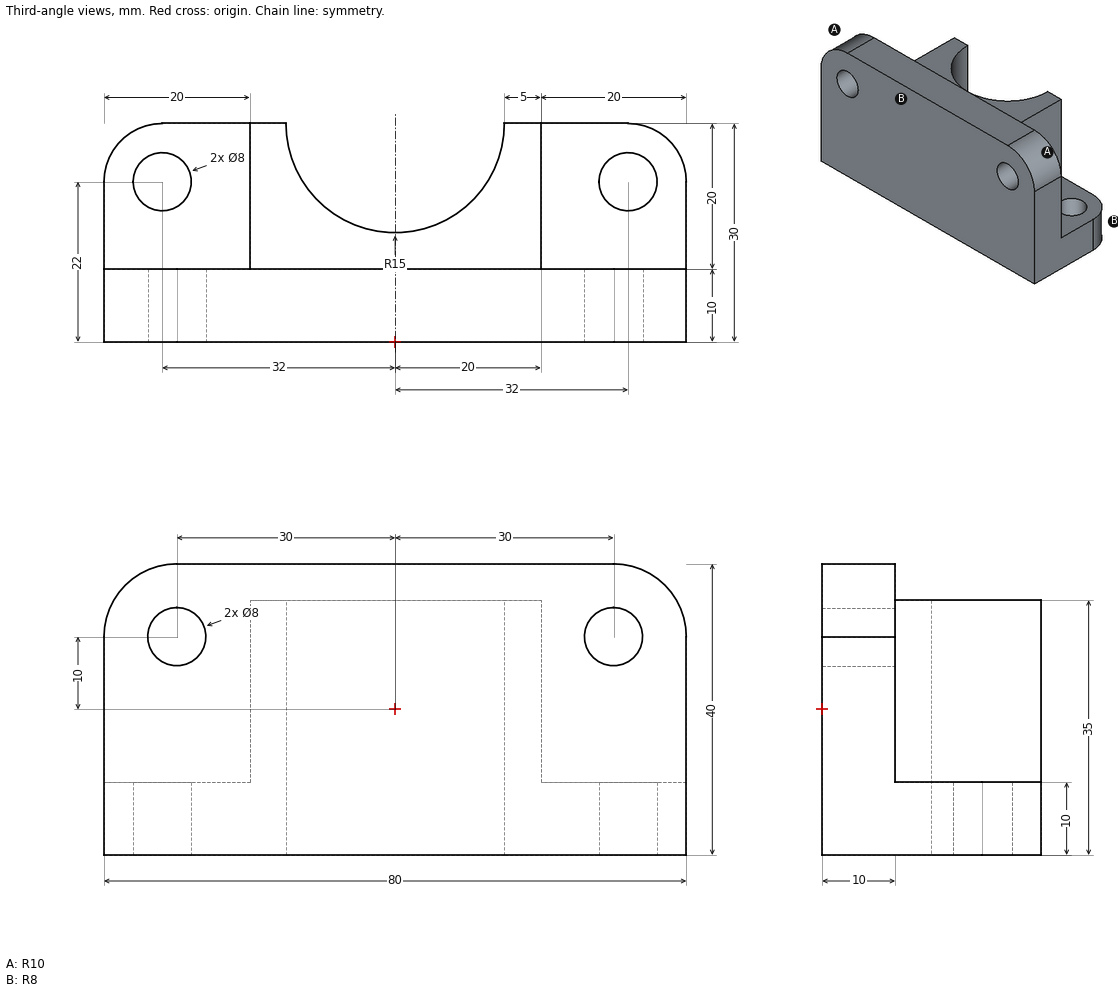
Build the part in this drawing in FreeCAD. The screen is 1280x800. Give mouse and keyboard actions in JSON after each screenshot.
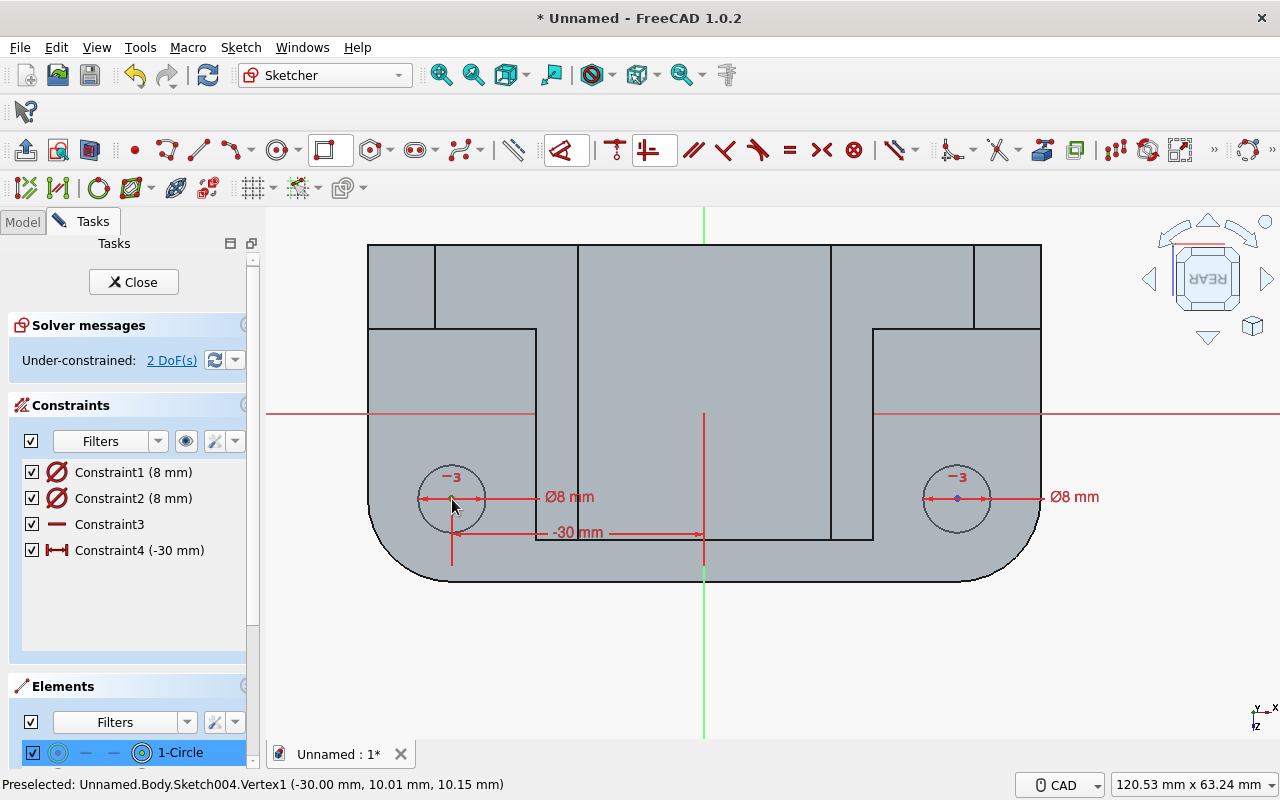
{"action": "key", "text": "i"}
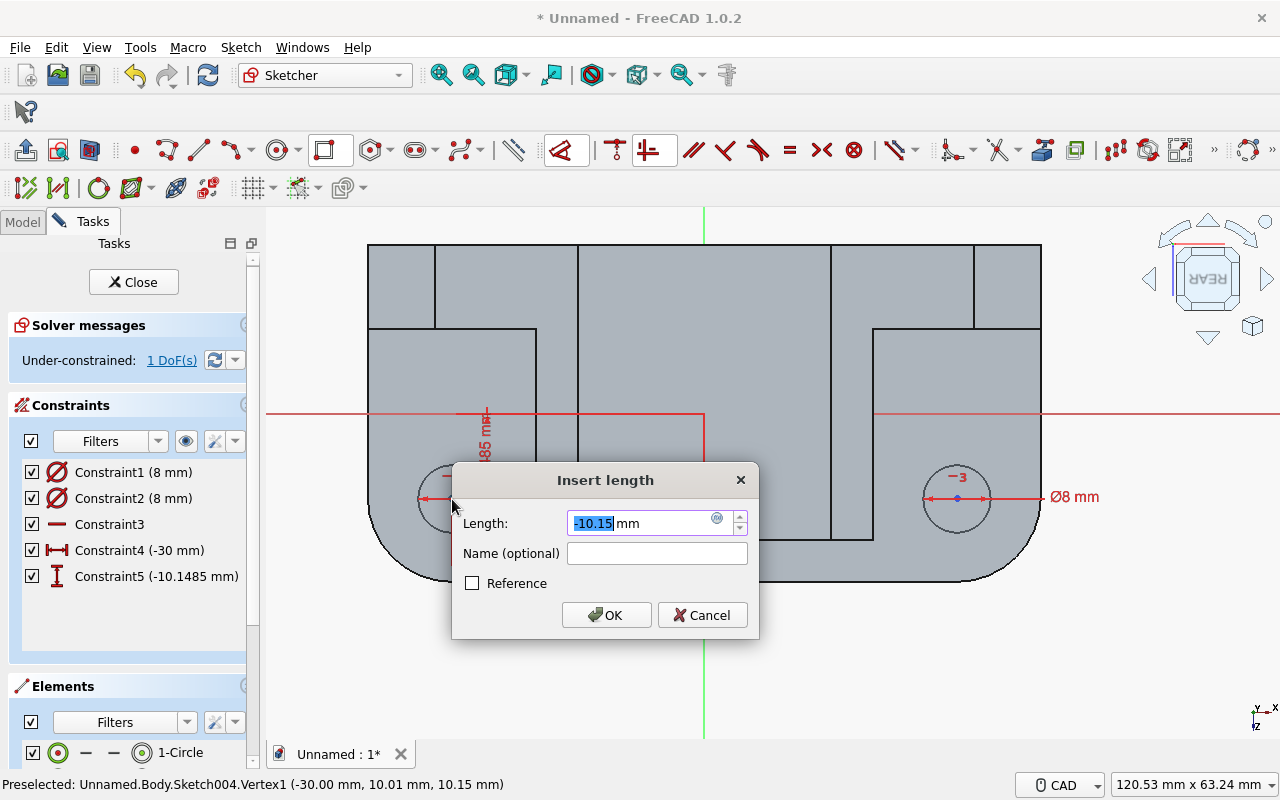
{"action": "type", "text": "-10"}
{"action": "key", "text": "Return"}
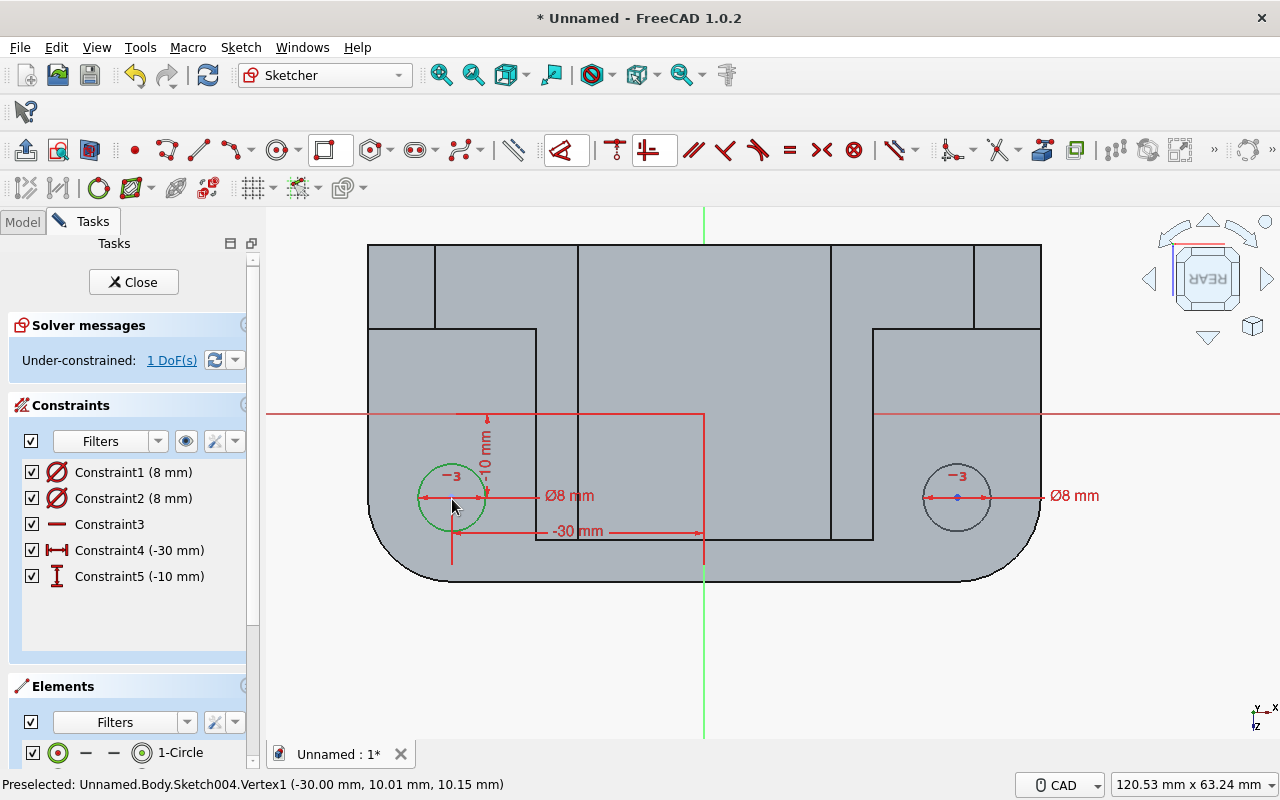
{"action": "left_click", "coordinate": [957, 498]}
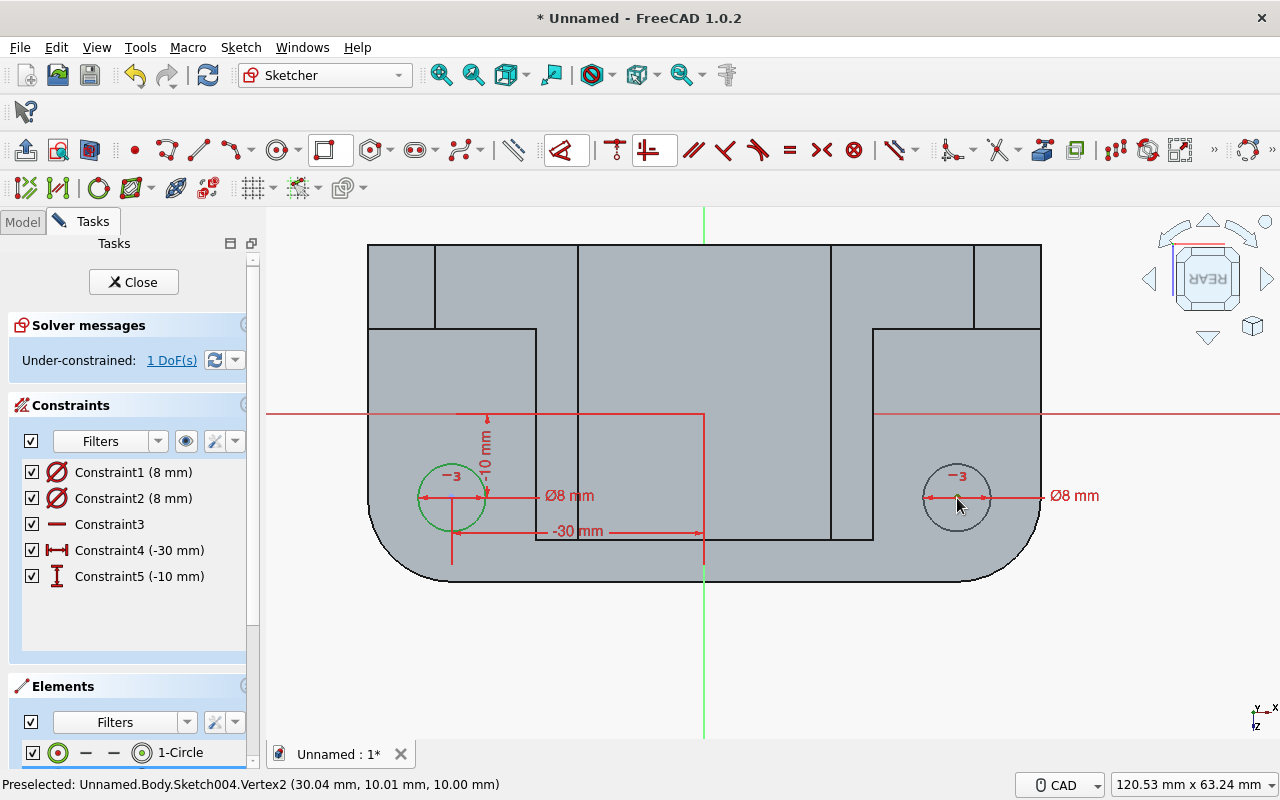
{"action": "key", "text": "l"}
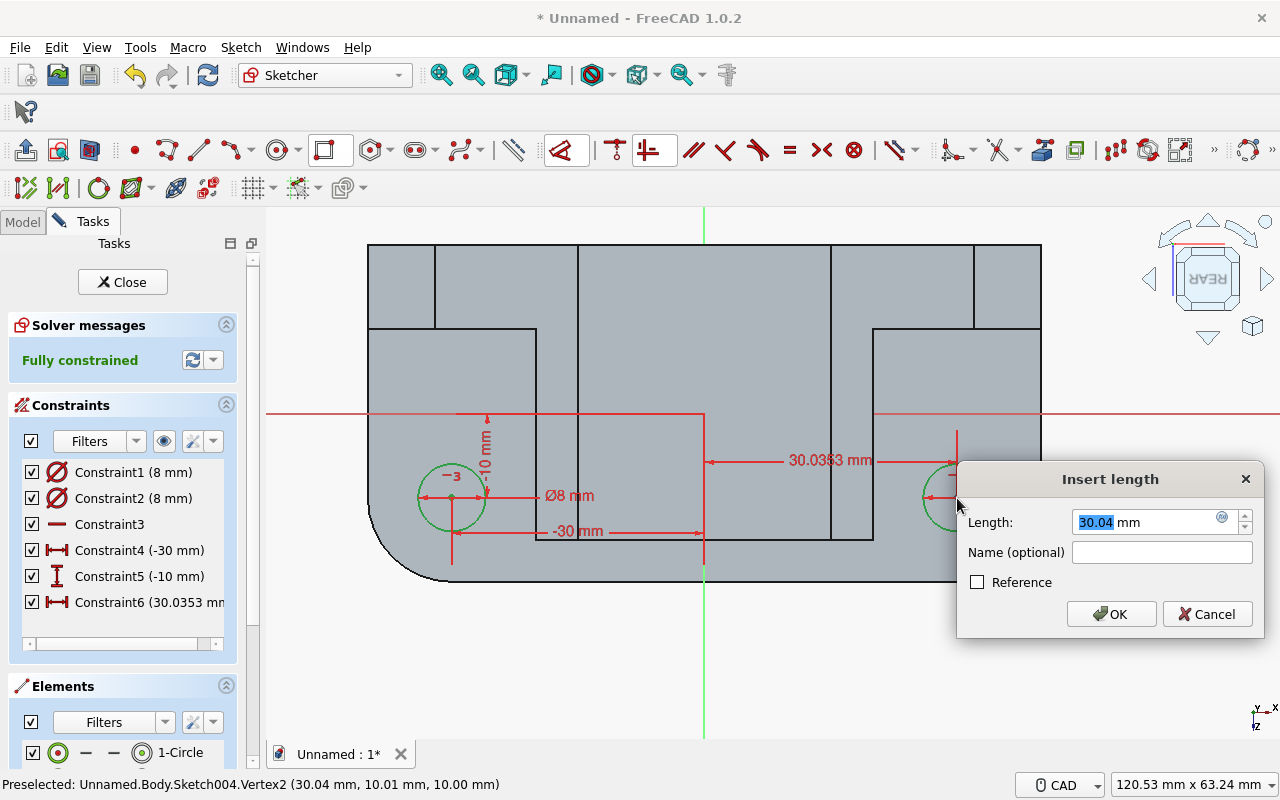
{"action": "type", "text": "30"}
{"action": "key", "text": "Return"}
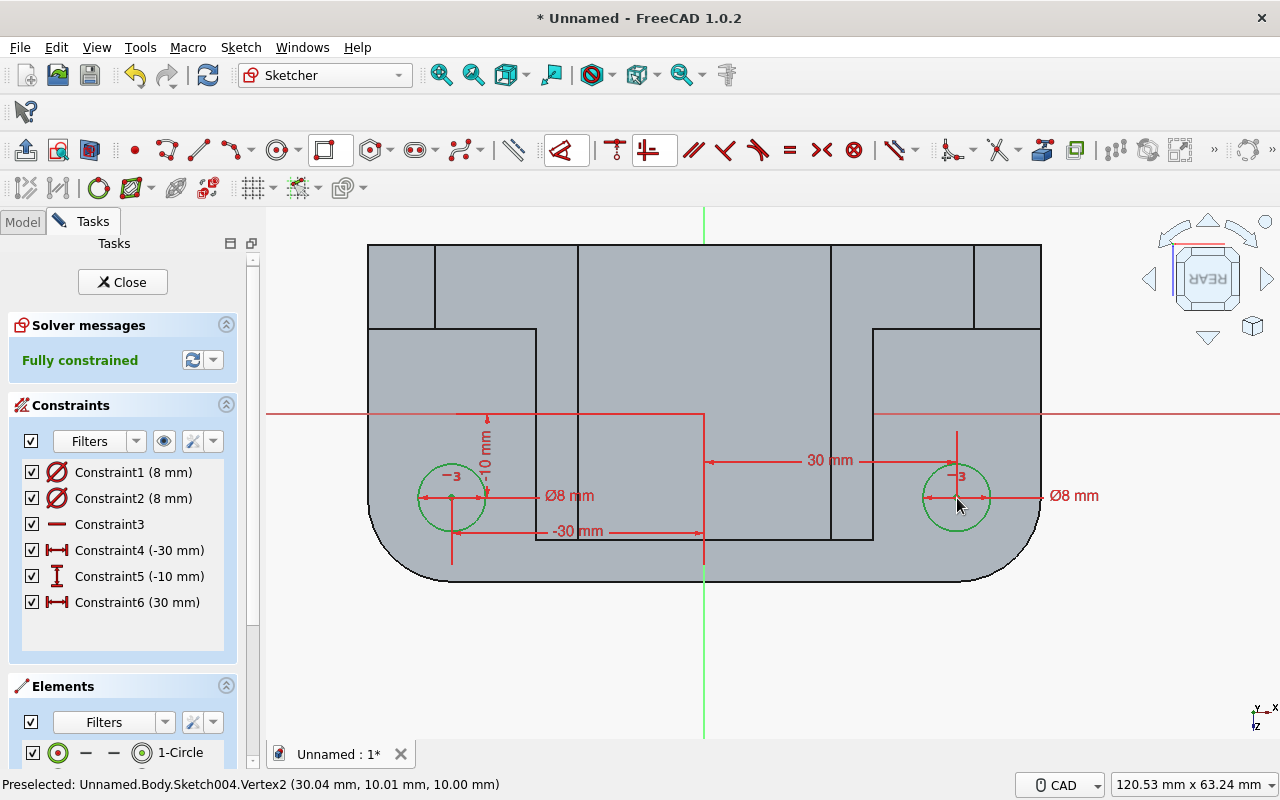
{"action": "left_click", "coordinate": [123, 282]}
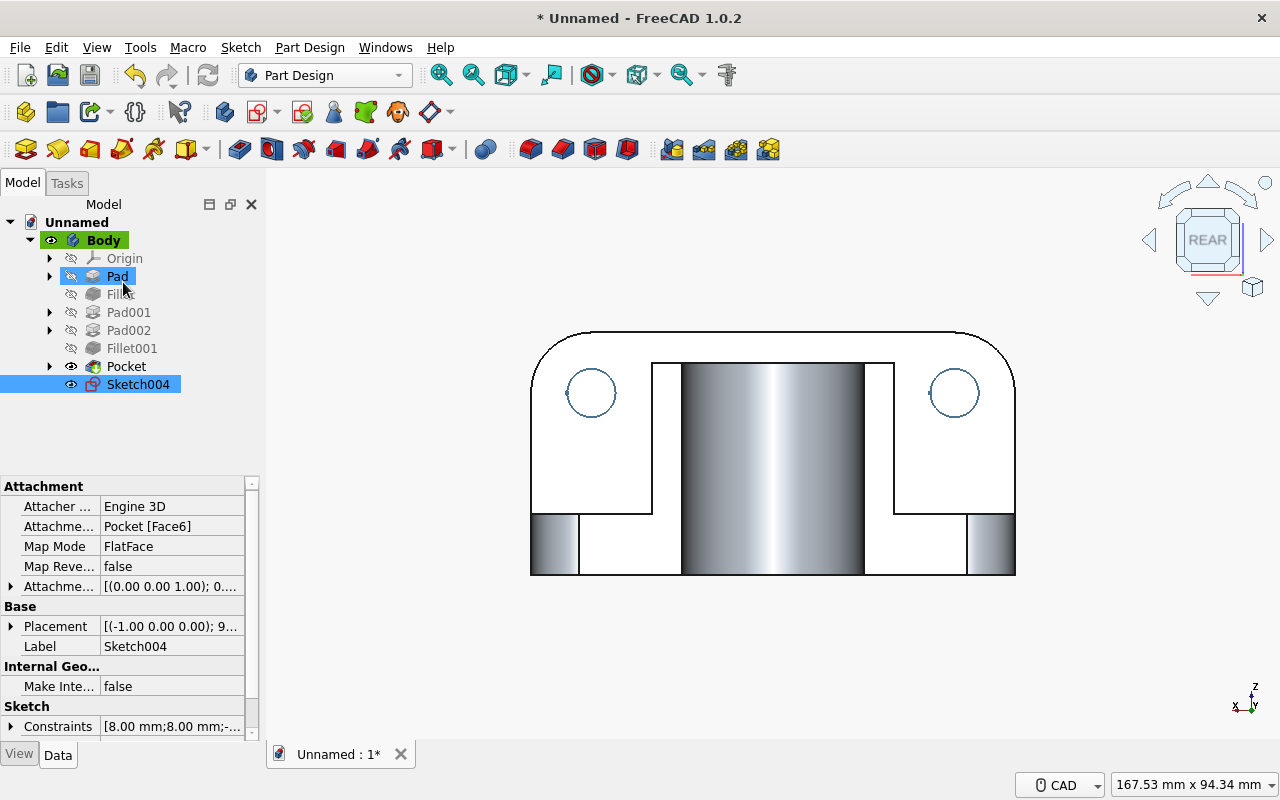
{"action": "left_click", "coordinate": [240, 150]}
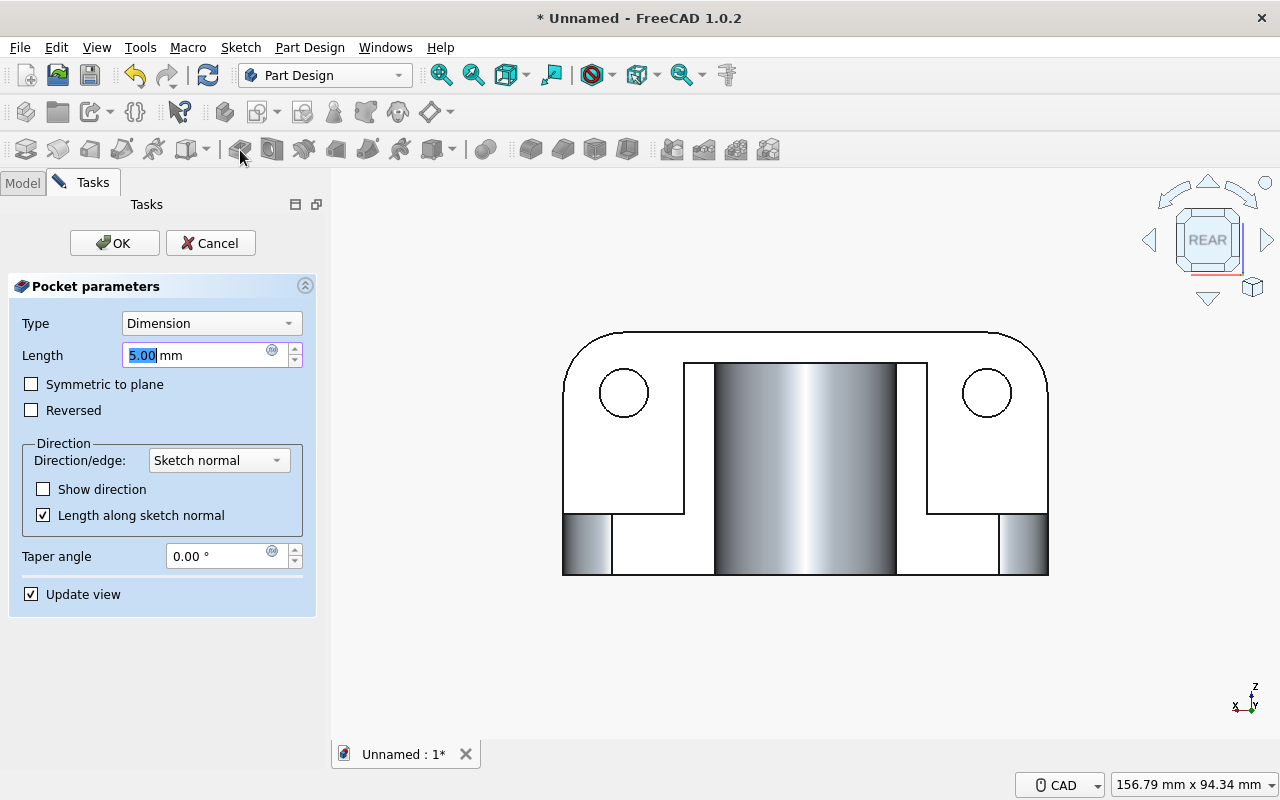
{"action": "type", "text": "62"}
{"action": "key", "text": "Tab"}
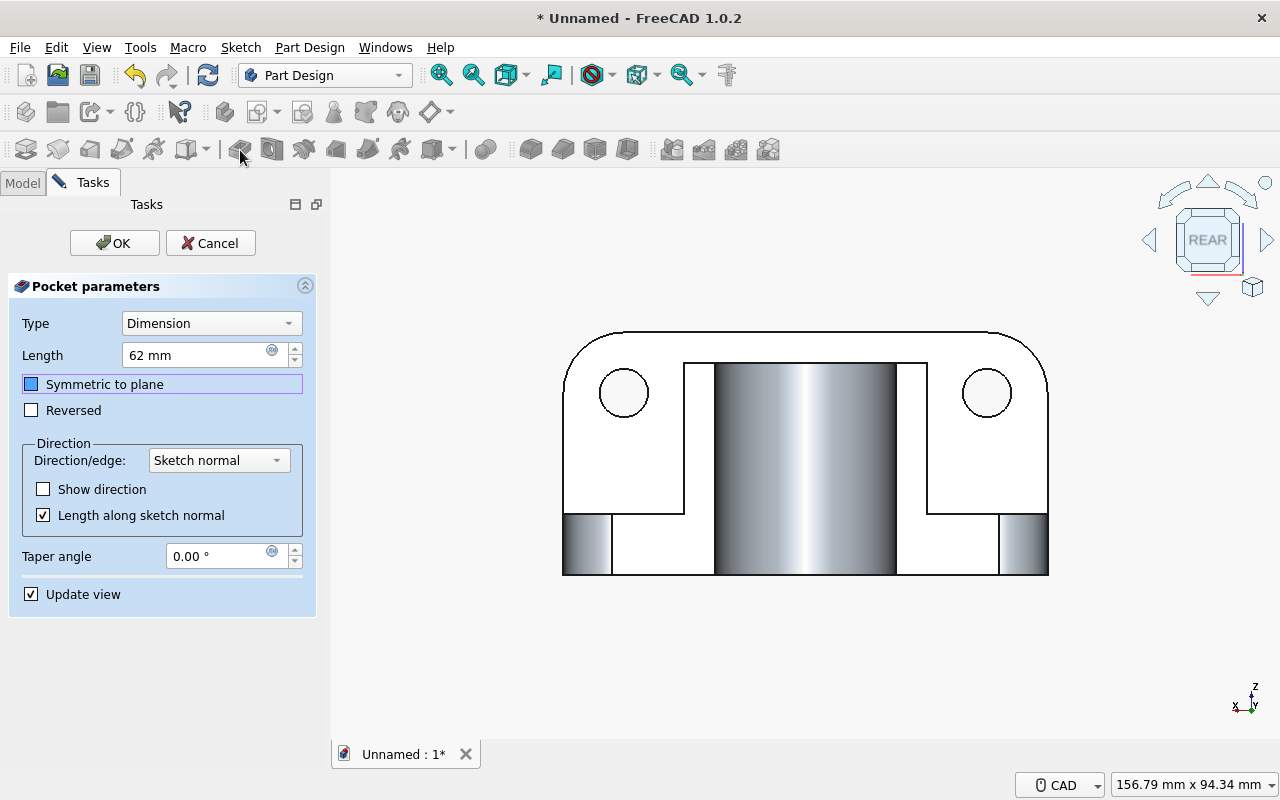
{"action": "left_click", "coordinate": [115, 243]}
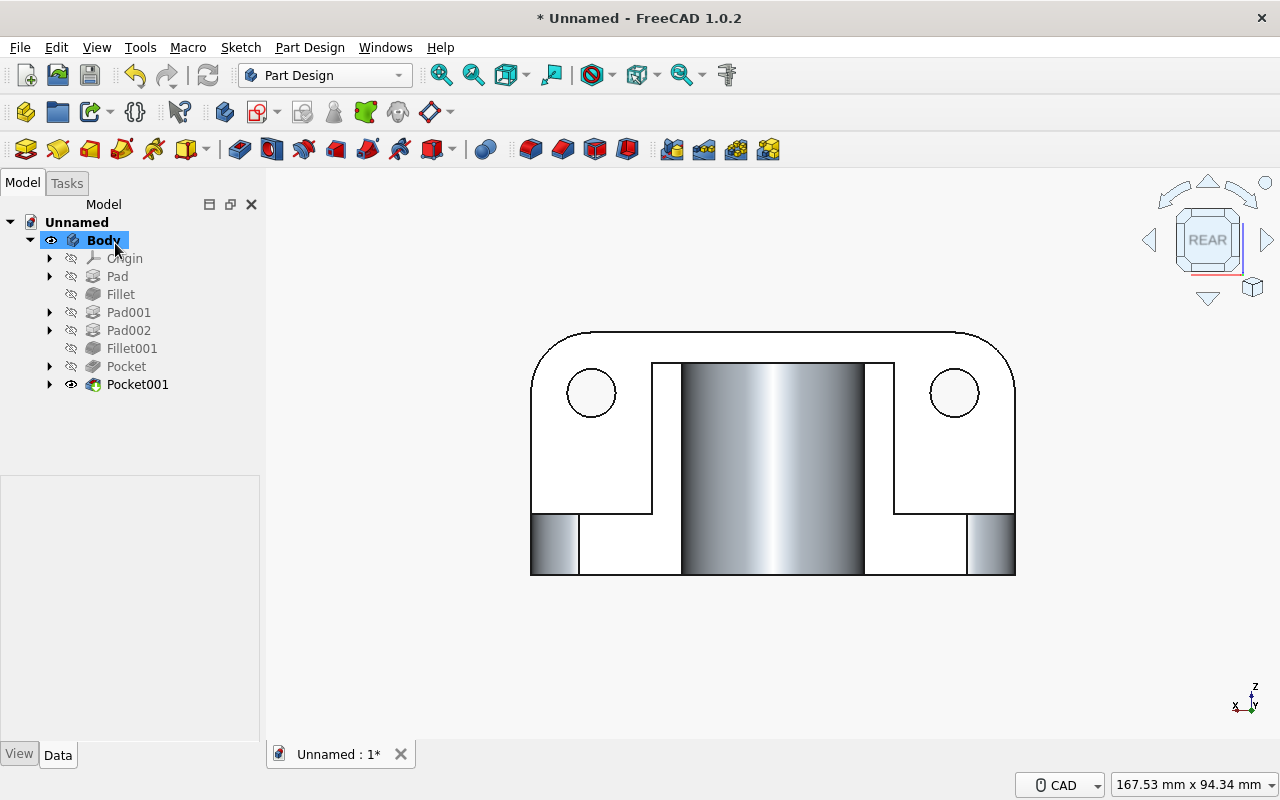
{"action": "key", "text": "0"}